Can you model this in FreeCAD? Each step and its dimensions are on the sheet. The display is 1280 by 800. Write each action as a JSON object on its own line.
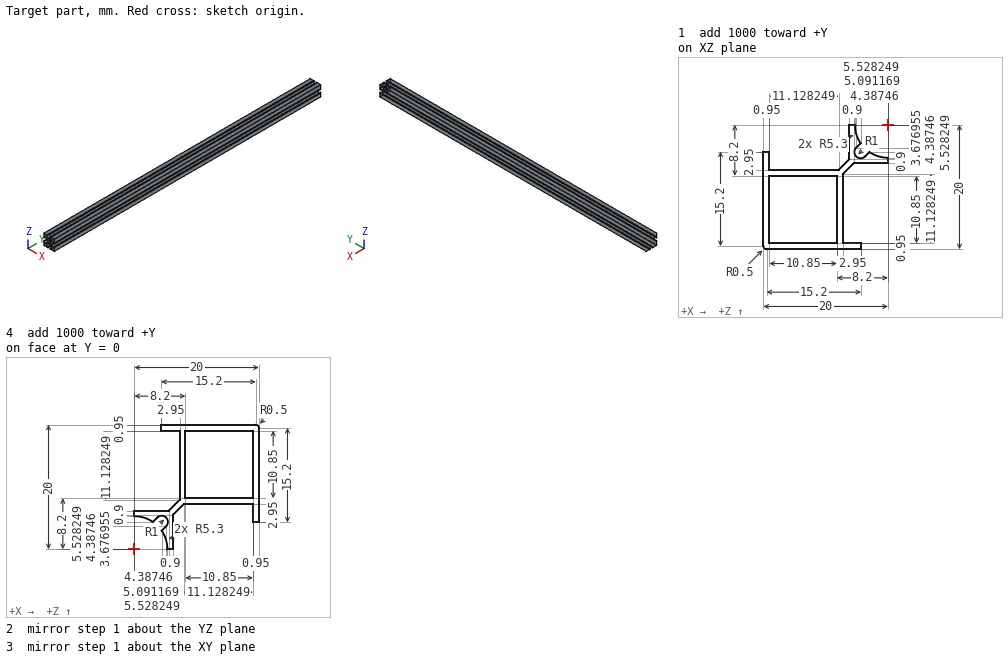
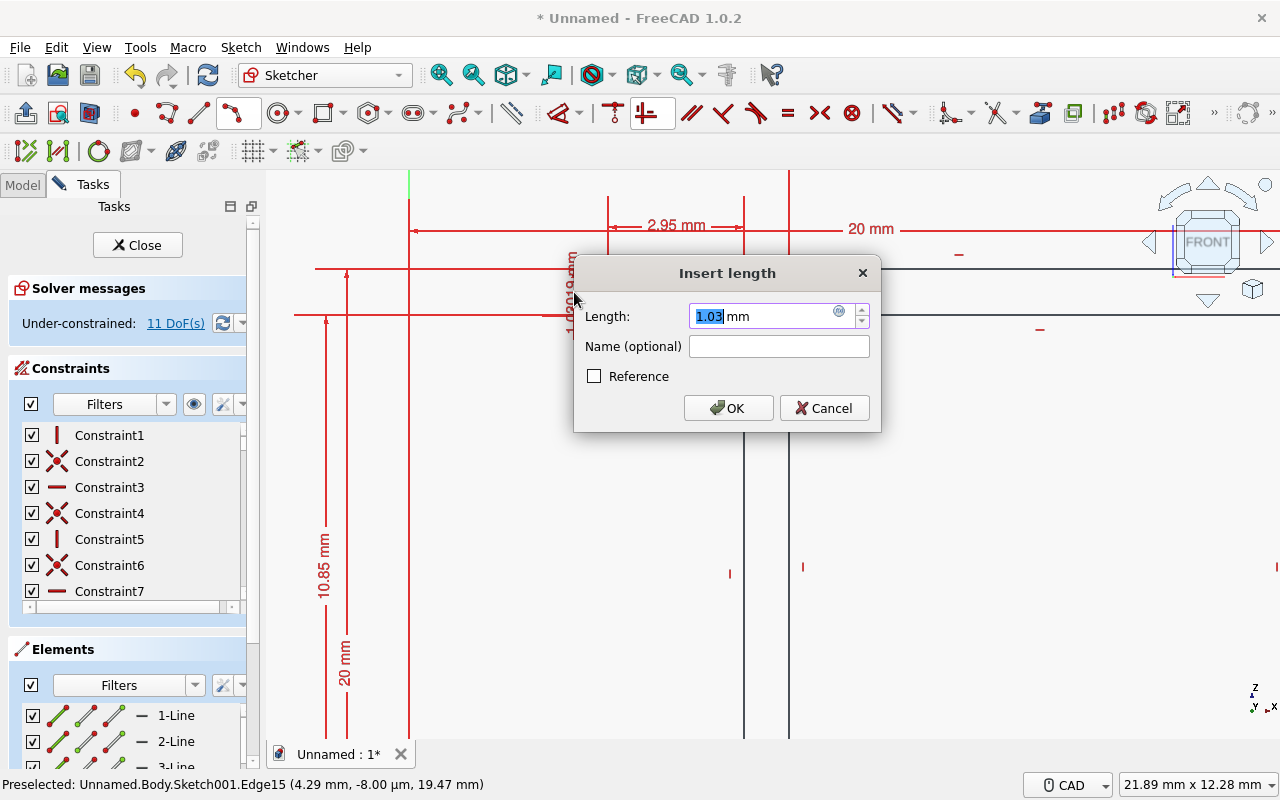
{"action": "type", "text": "0.95"}
{"action": "key", "text": "Return"}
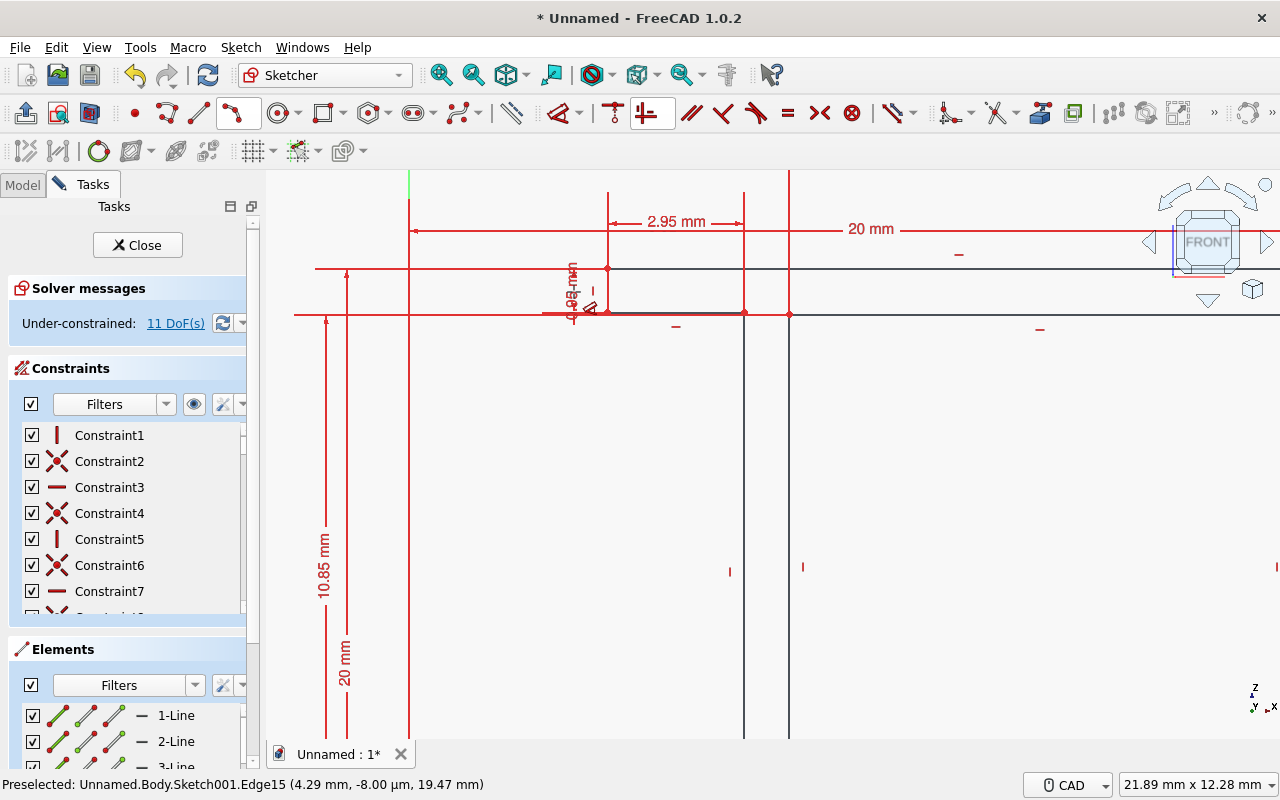
{"action": "scroll", "coordinate": [607, 293], "scroll_direction": "down", "scroll_amount": 5}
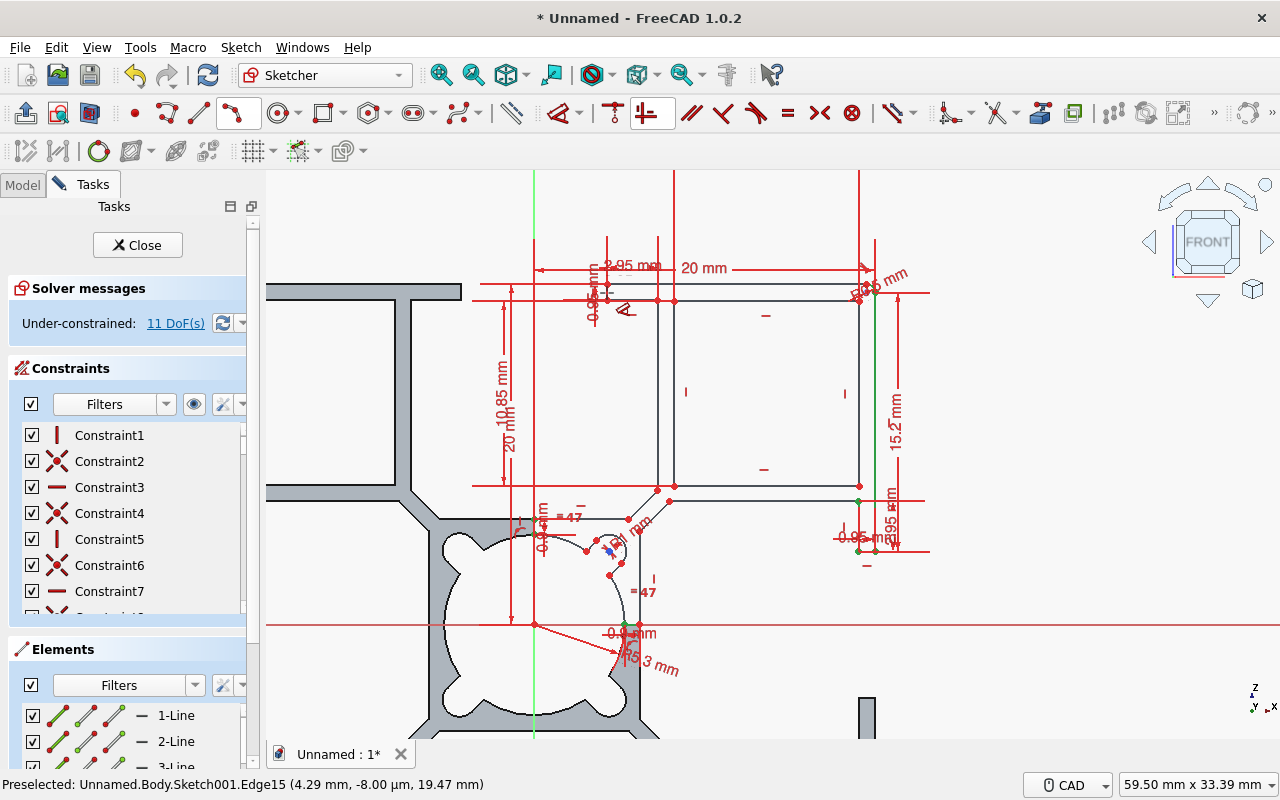
{"action": "left_click", "coordinate": [685, 284]}
{"action": "left_click", "coordinate": [737, 250]}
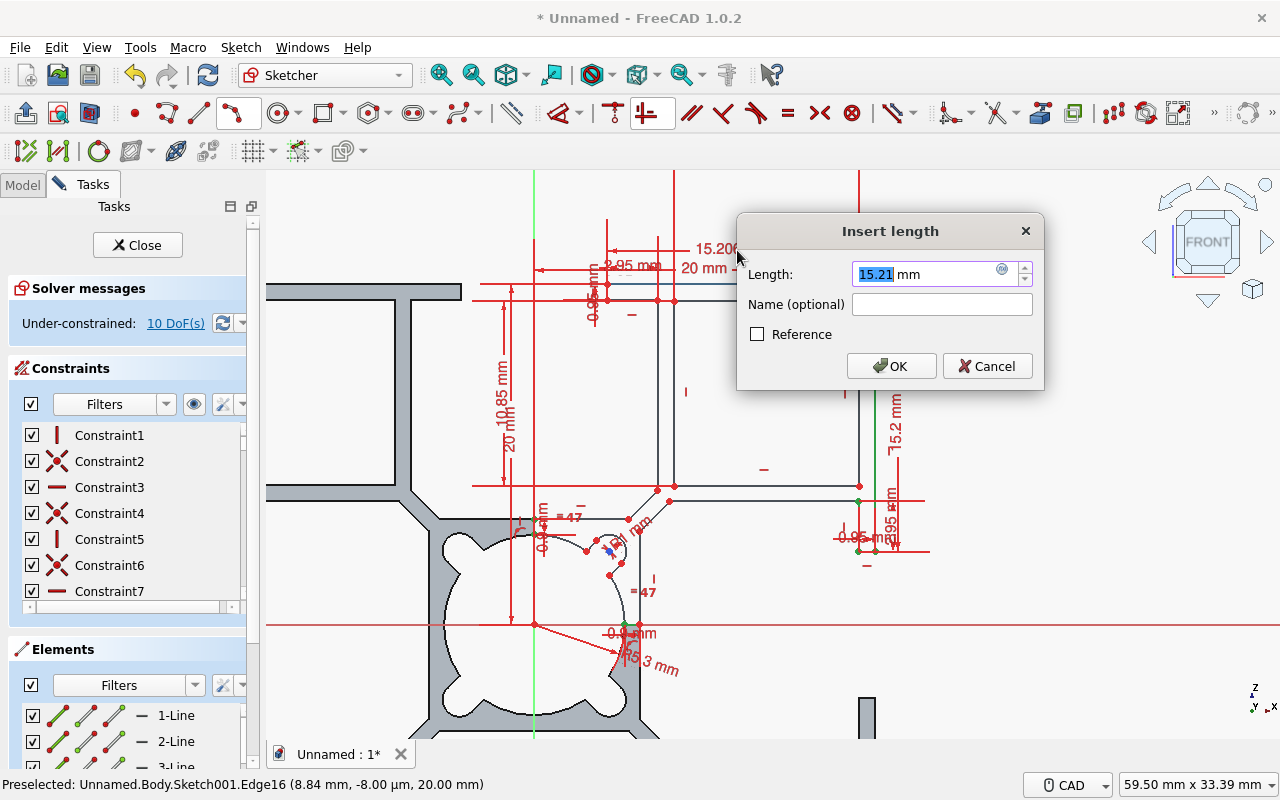
{"action": "type", "text": "15.2"}
{"action": "key", "text": "Return"}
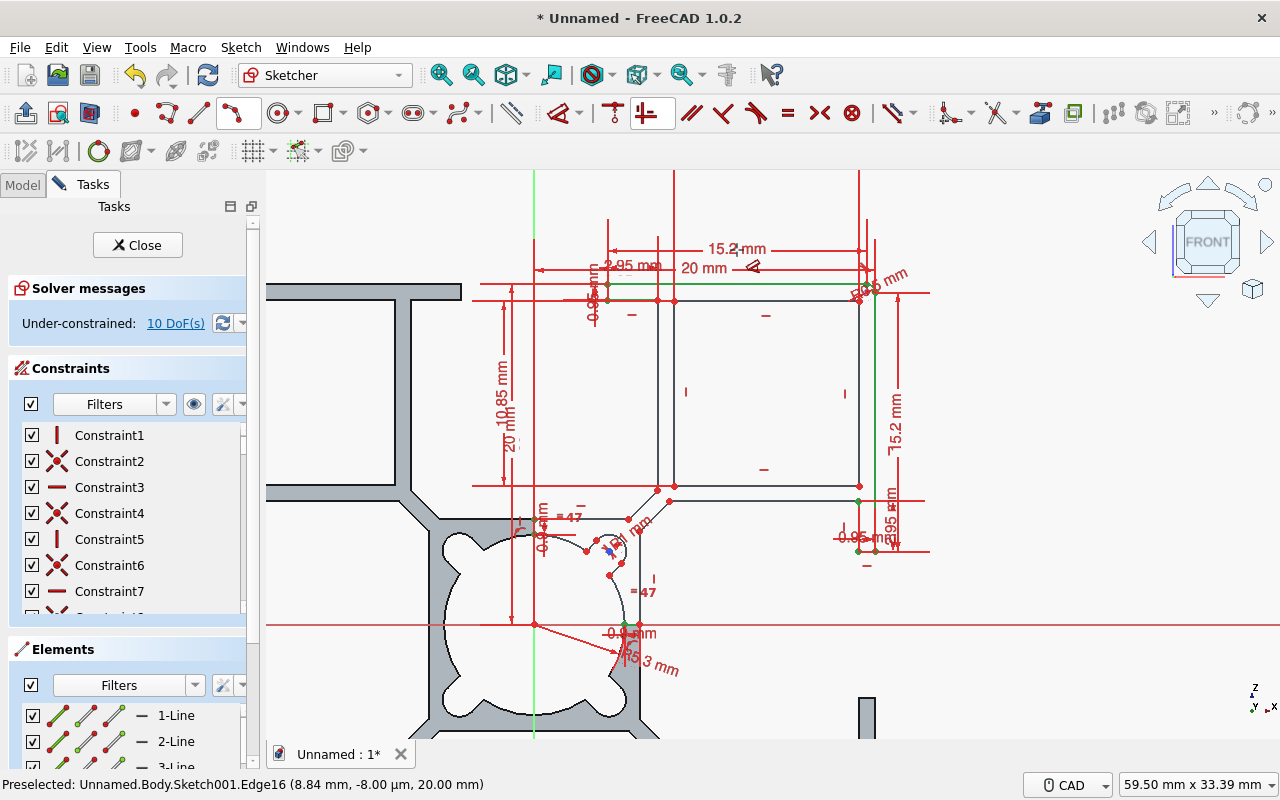
{"action": "left_click", "coordinate": [674, 301]}
{"action": "left_click", "coordinate": [572, 659]}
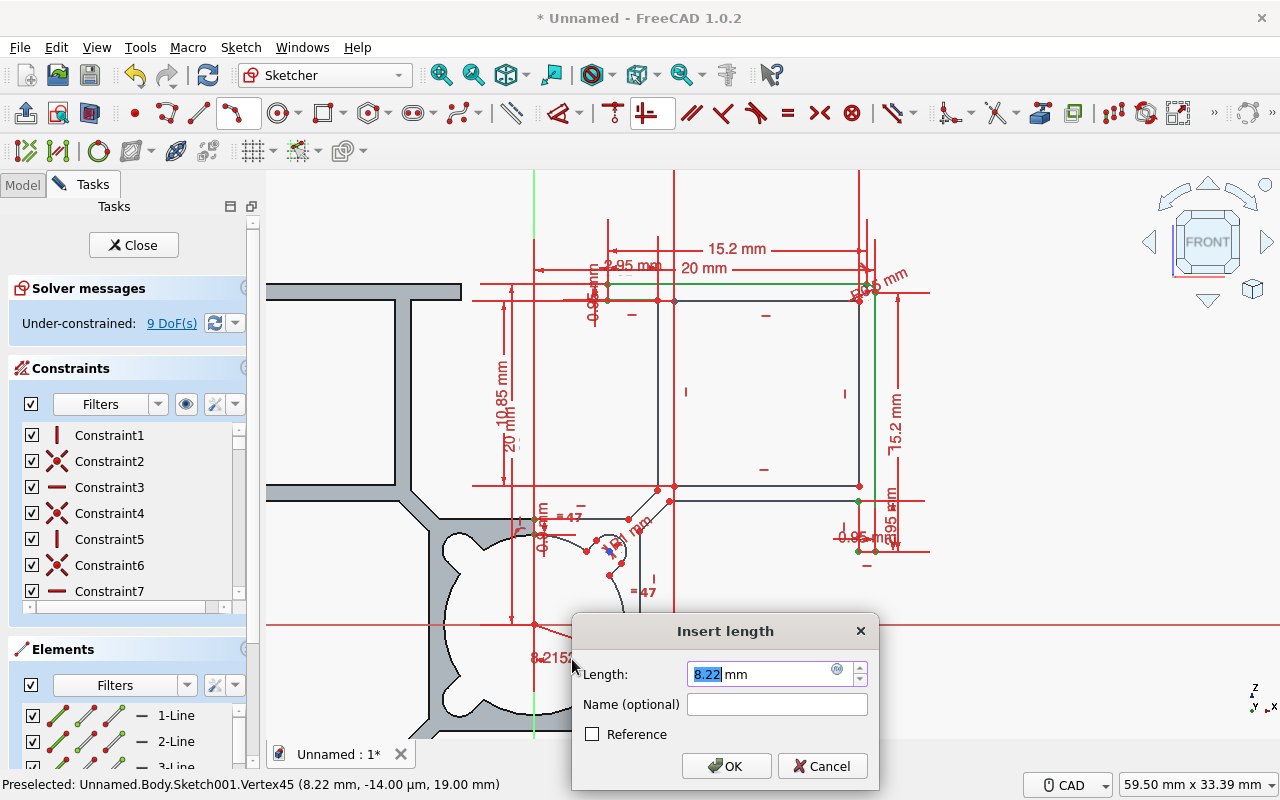
{"action": "type", "text": "8.2"}
{"action": "key", "text": "Return"}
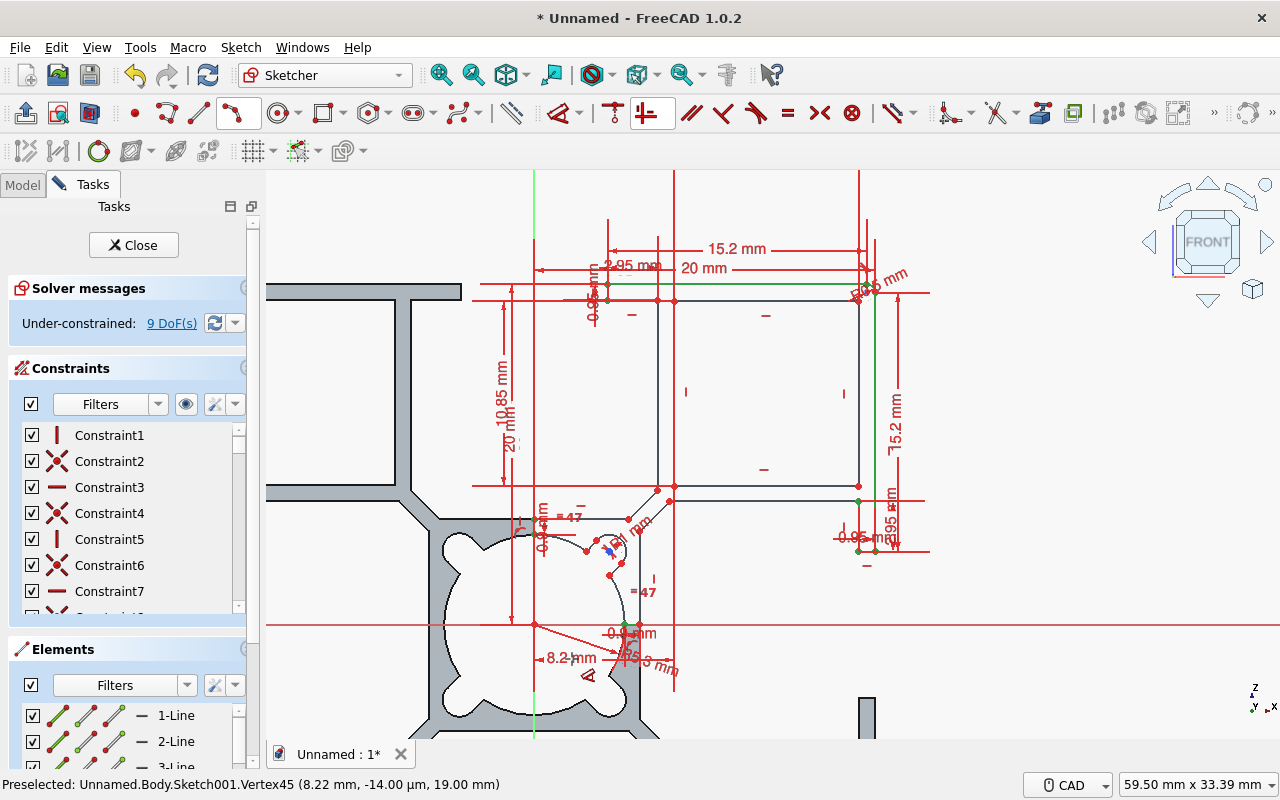
{"action": "left_click", "coordinate": [674, 486]}
{"action": "left_click", "coordinate": [500, 556]}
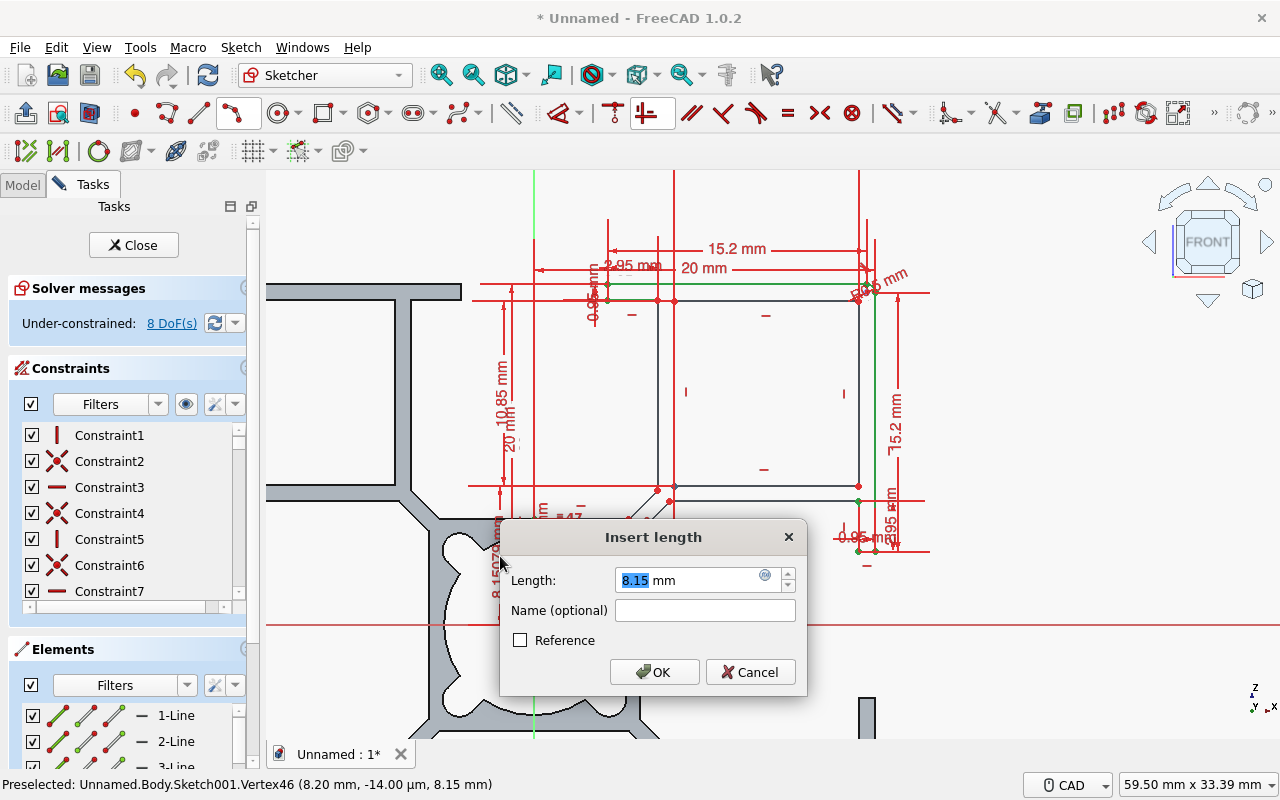
{"action": "type", "text": "8.2"}
{"action": "key", "text": "Return"}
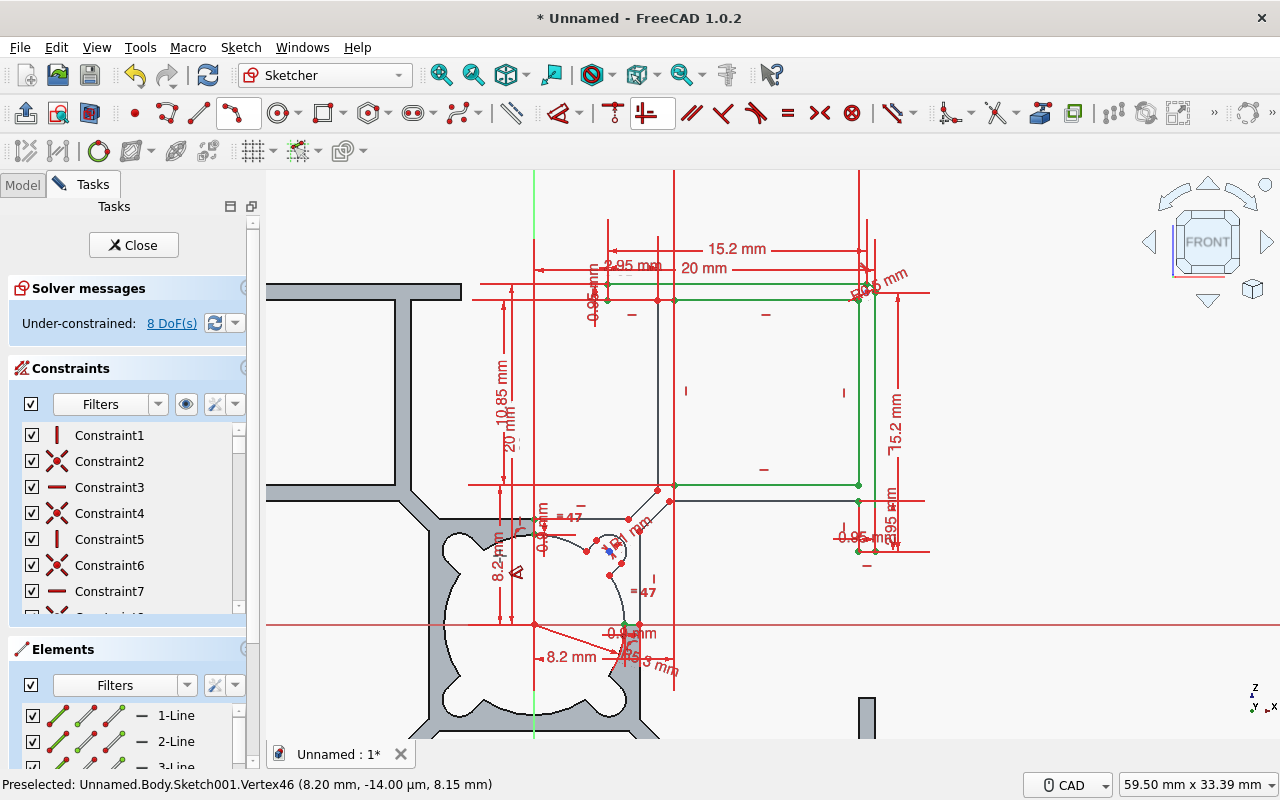
{"action": "left_click", "coordinate": [640, 560]}
{"action": "left_click", "coordinate": [606, 557]}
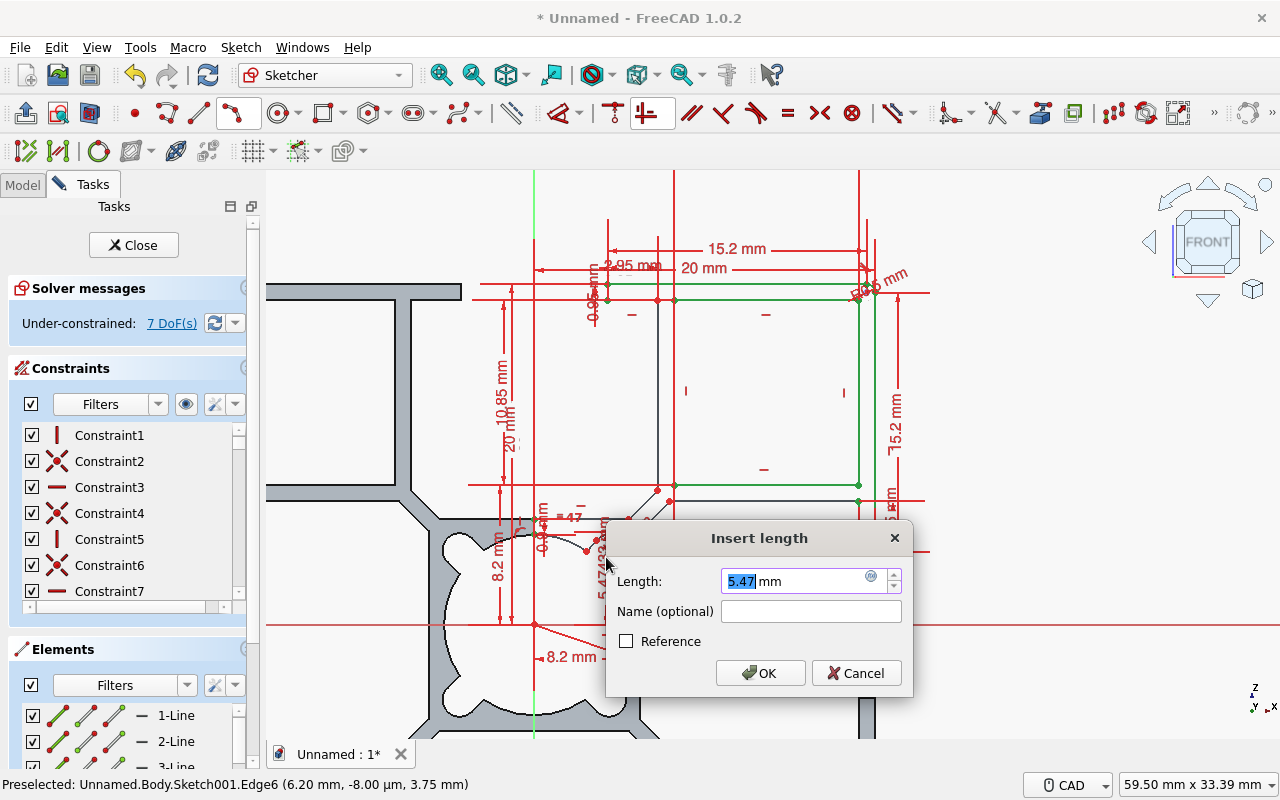
{"action": "type", "text": "5.528249"}
{"action": "key", "text": "Return"}